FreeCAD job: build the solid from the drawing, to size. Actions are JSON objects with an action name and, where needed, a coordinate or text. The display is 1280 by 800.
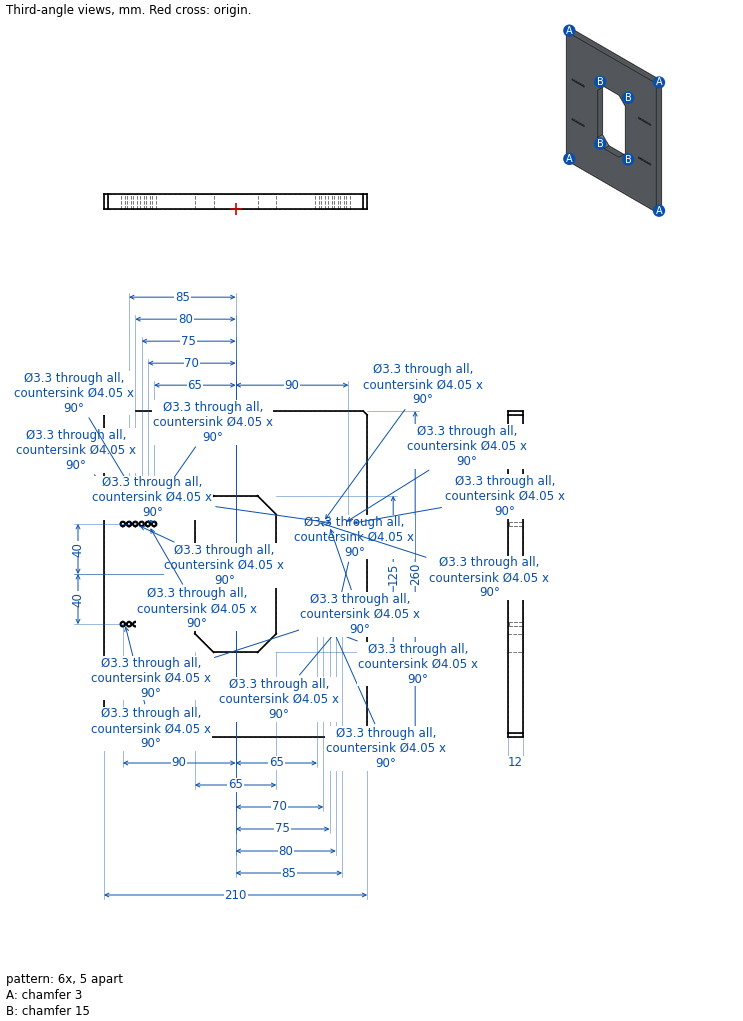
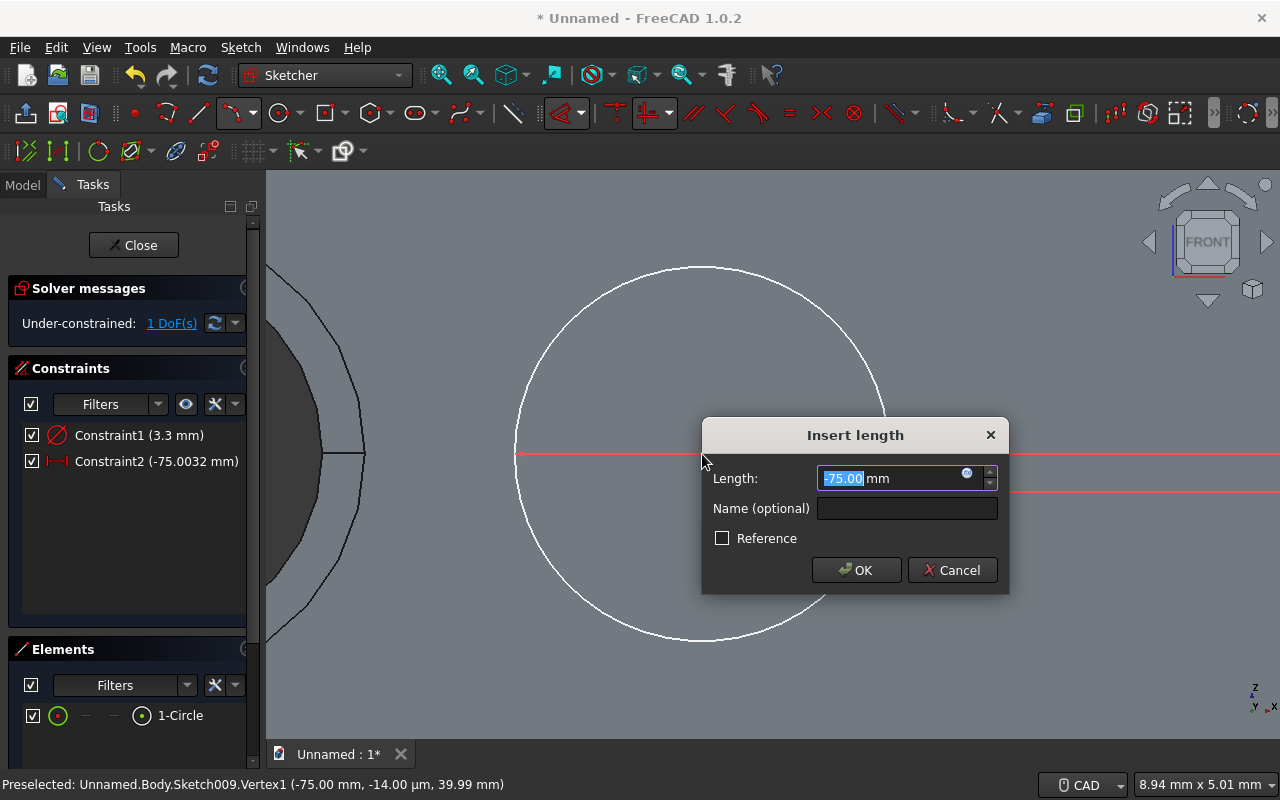
{"action": "type", "text": "-75"}
{"action": "key", "text": "Return"}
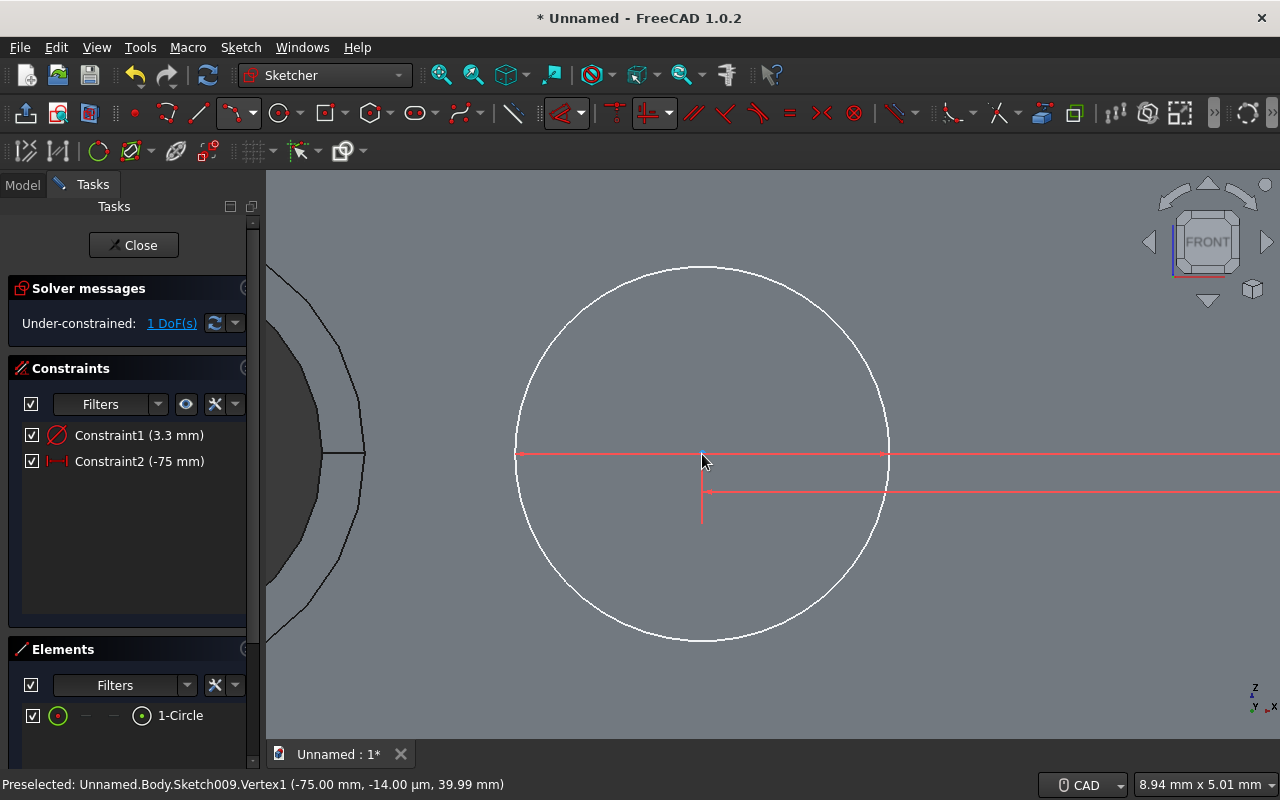
{"action": "left_click", "coordinate": [702, 454]}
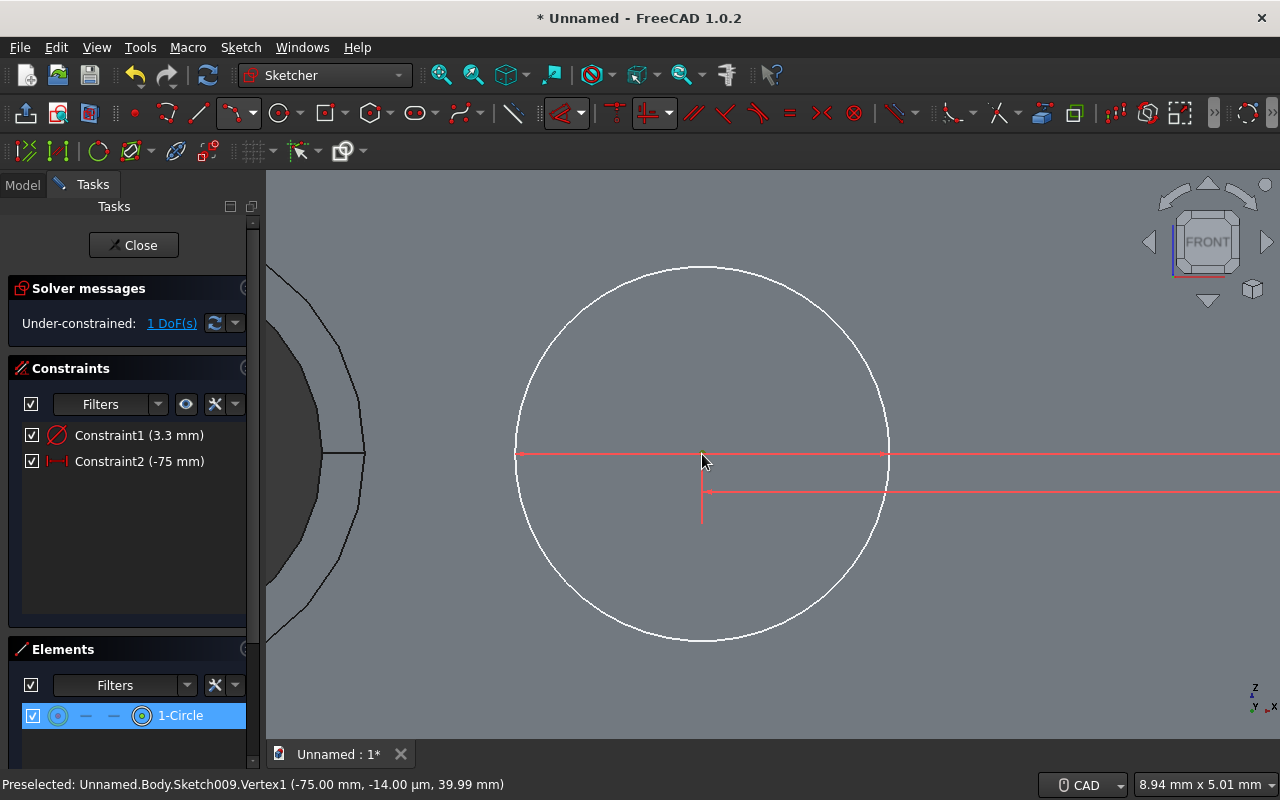
{"action": "key", "text": "i"}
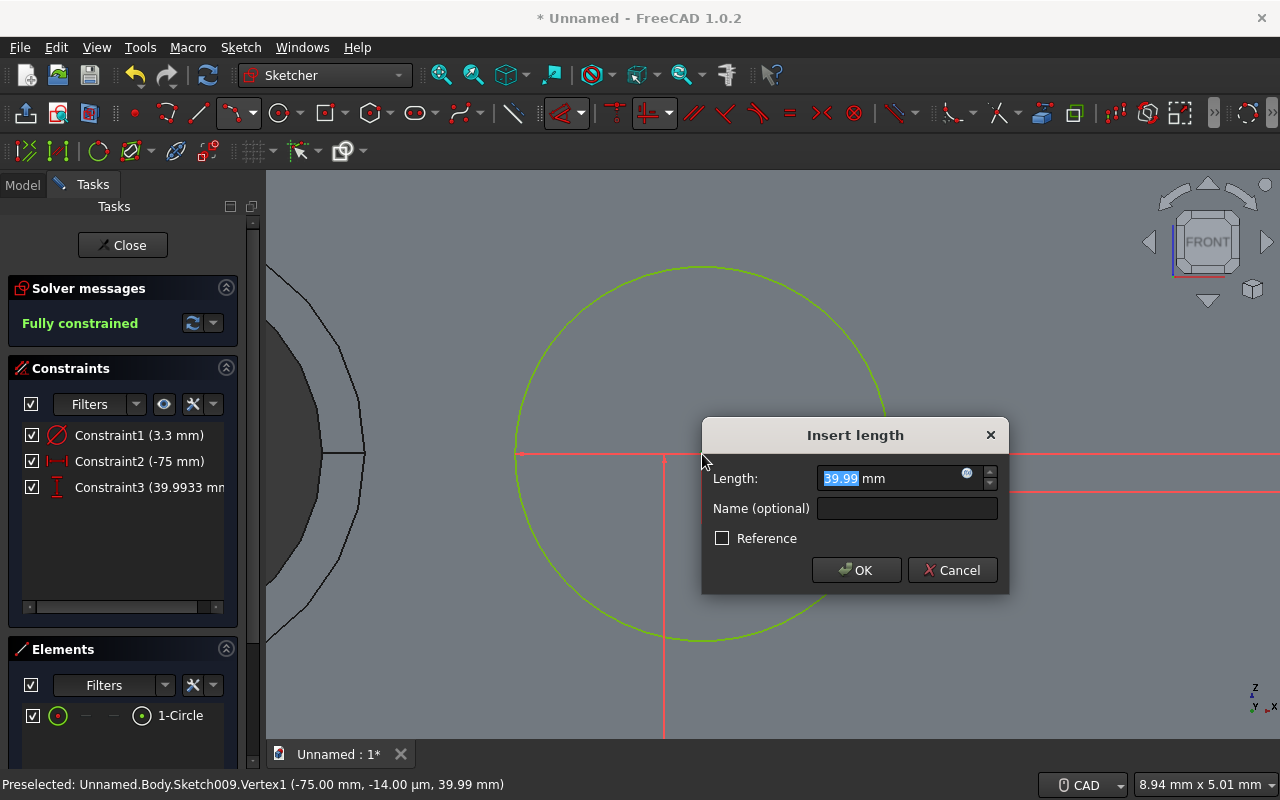
{"action": "type", "text": "40"}
{"action": "key", "text": "Return"}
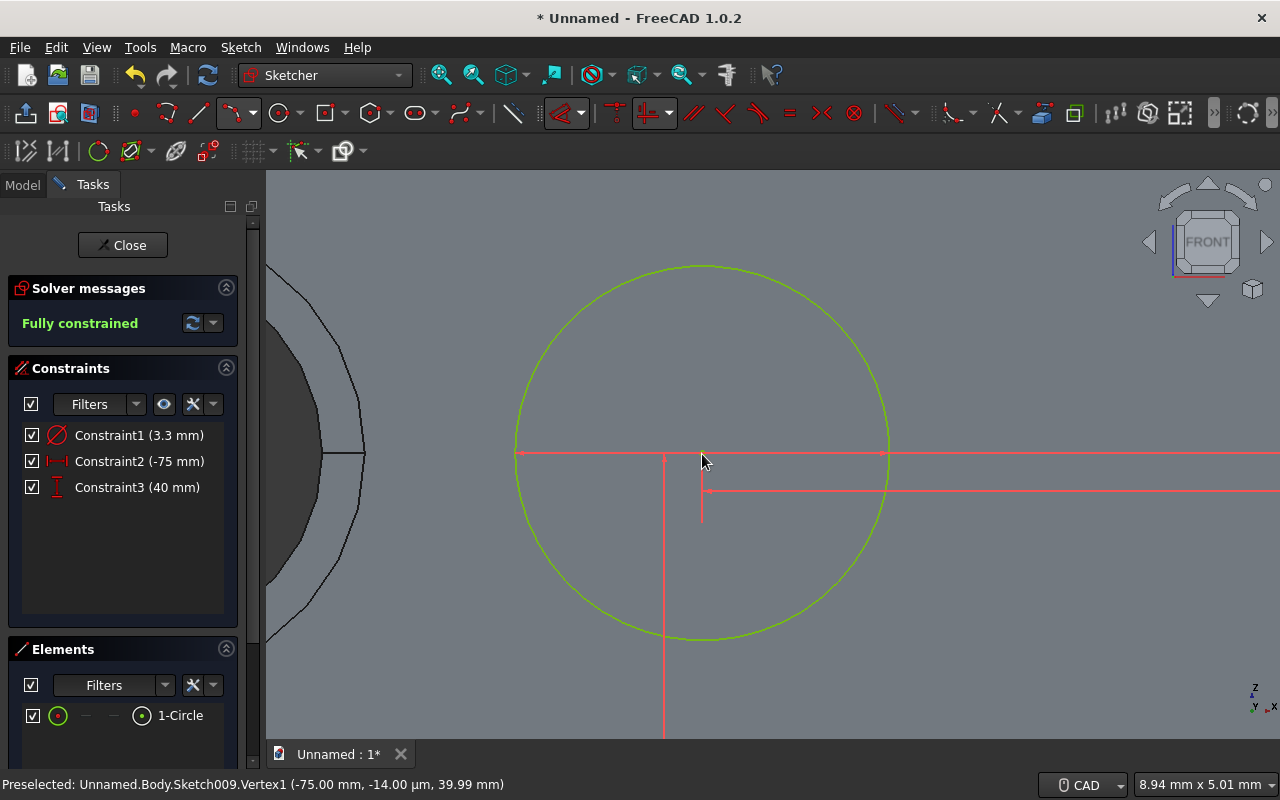
{"action": "left_click", "coordinate": [123, 245]}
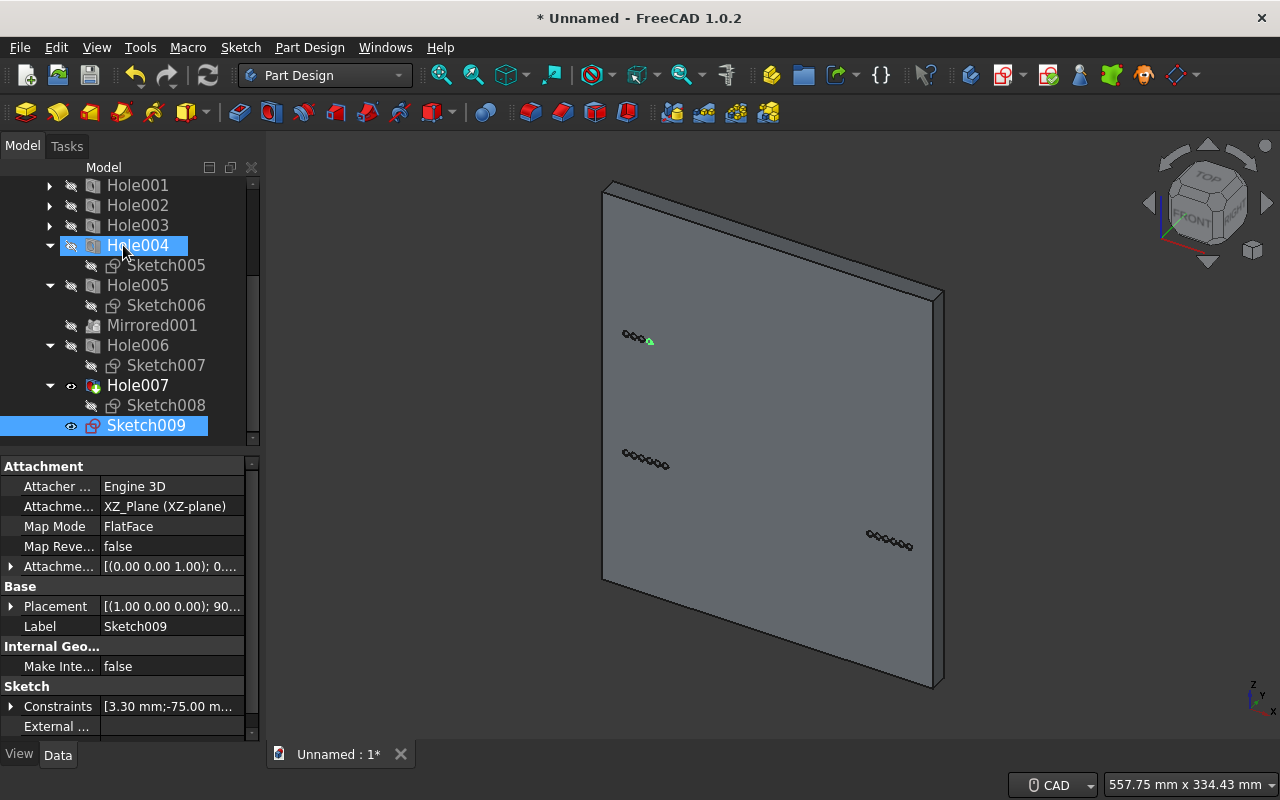
{"action": "left_click", "coordinate": [272, 112]}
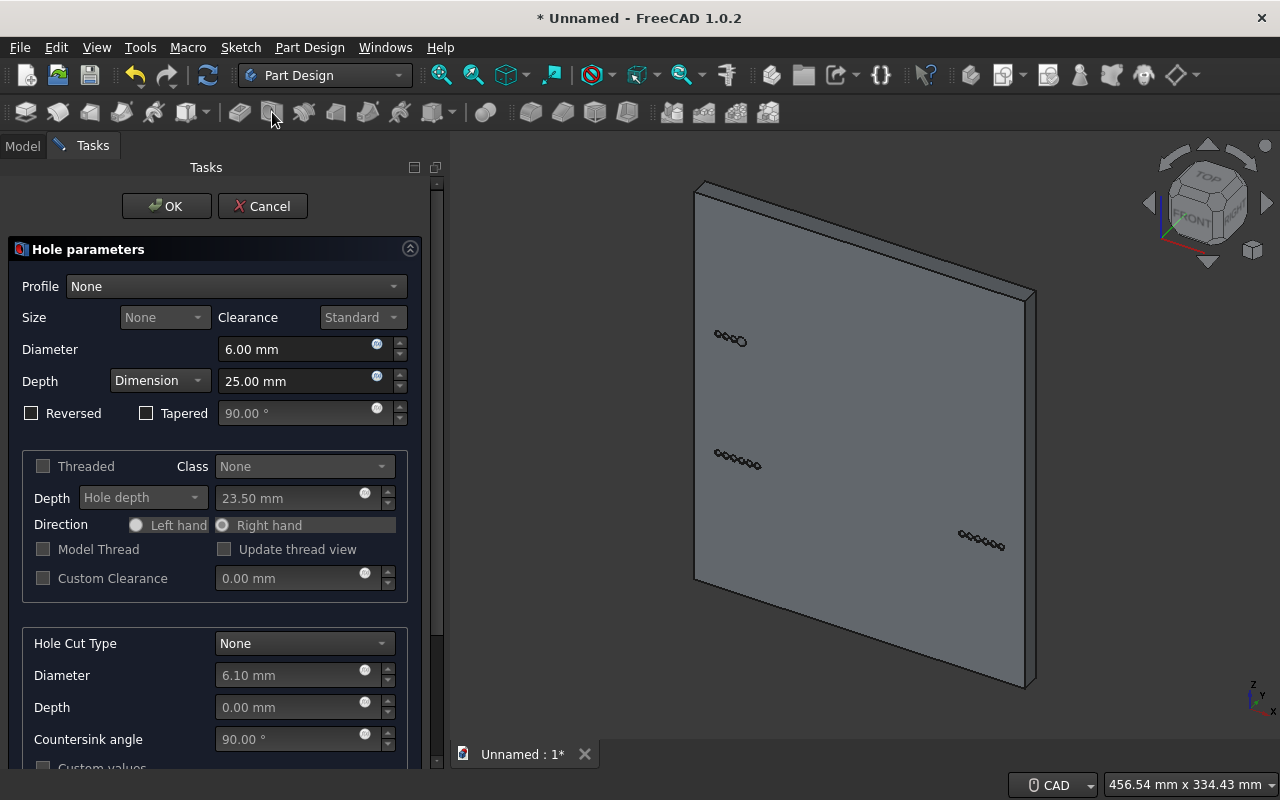
{"action": "triple_click", "coordinate": [305, 349]}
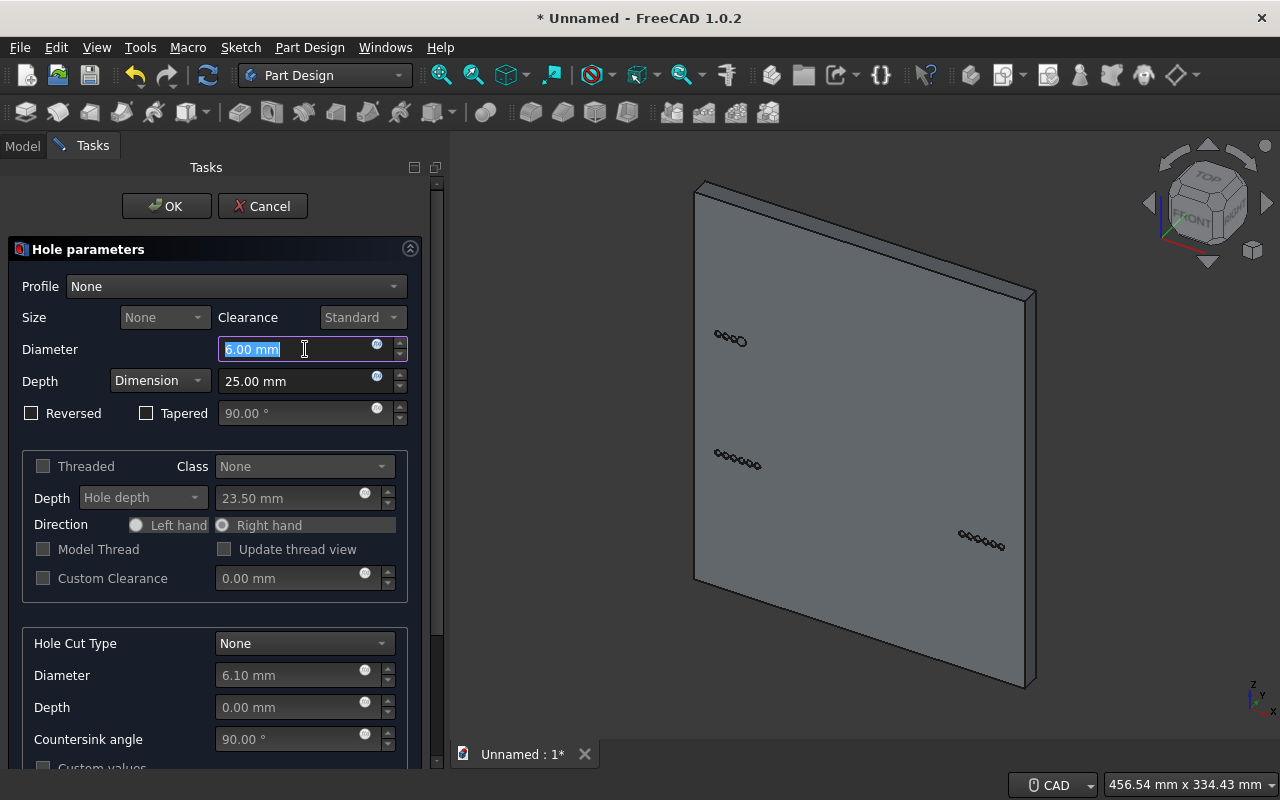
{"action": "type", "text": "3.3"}
{"action": "key", "text": "Tab"}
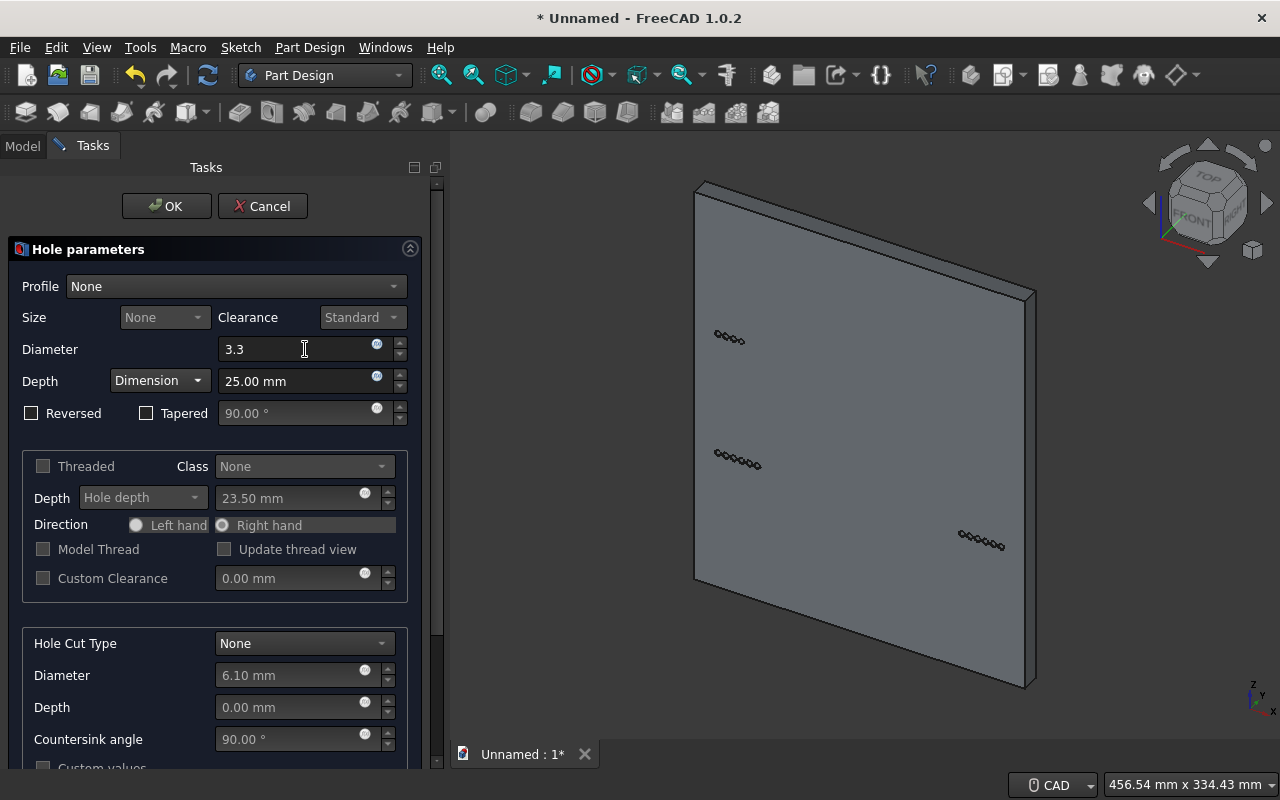
{"action": "left_click", "coordinate": [161, 380]}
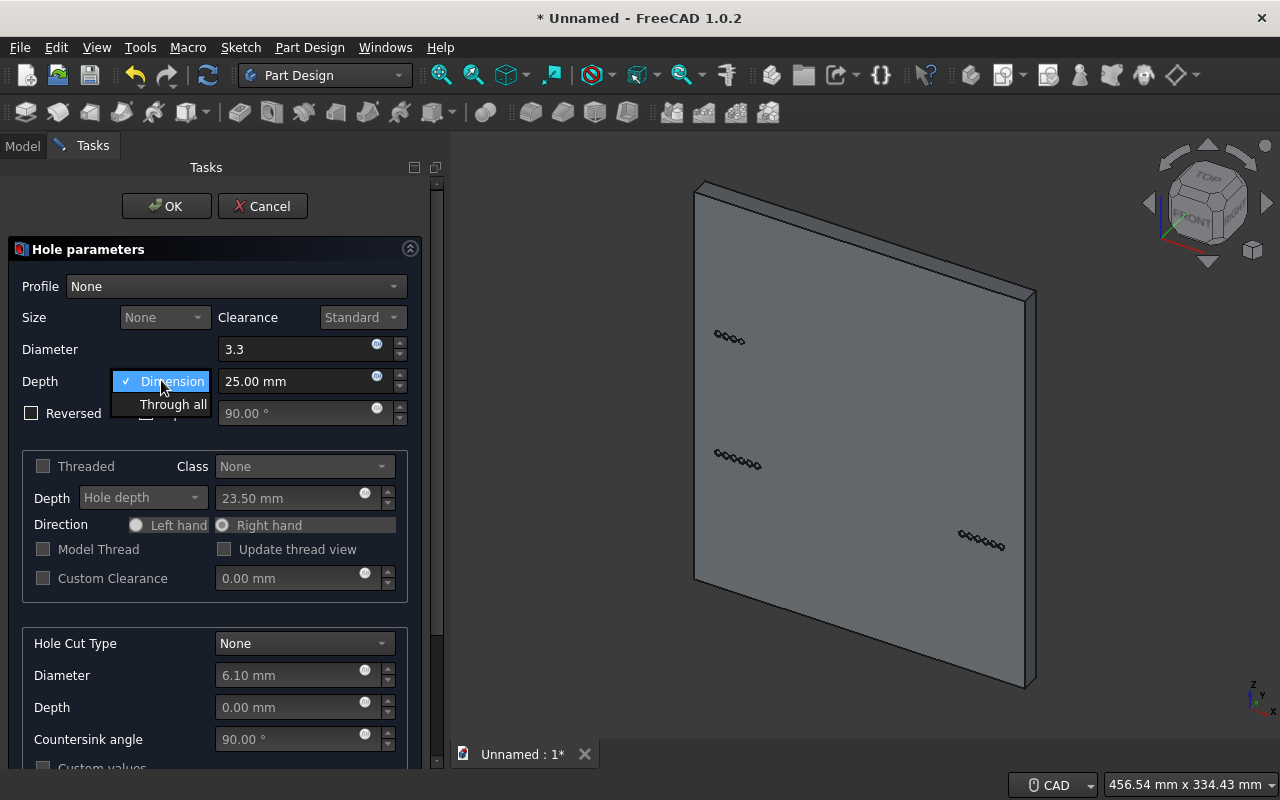
{"action": "left_click", "coordinate": [160, 404]}